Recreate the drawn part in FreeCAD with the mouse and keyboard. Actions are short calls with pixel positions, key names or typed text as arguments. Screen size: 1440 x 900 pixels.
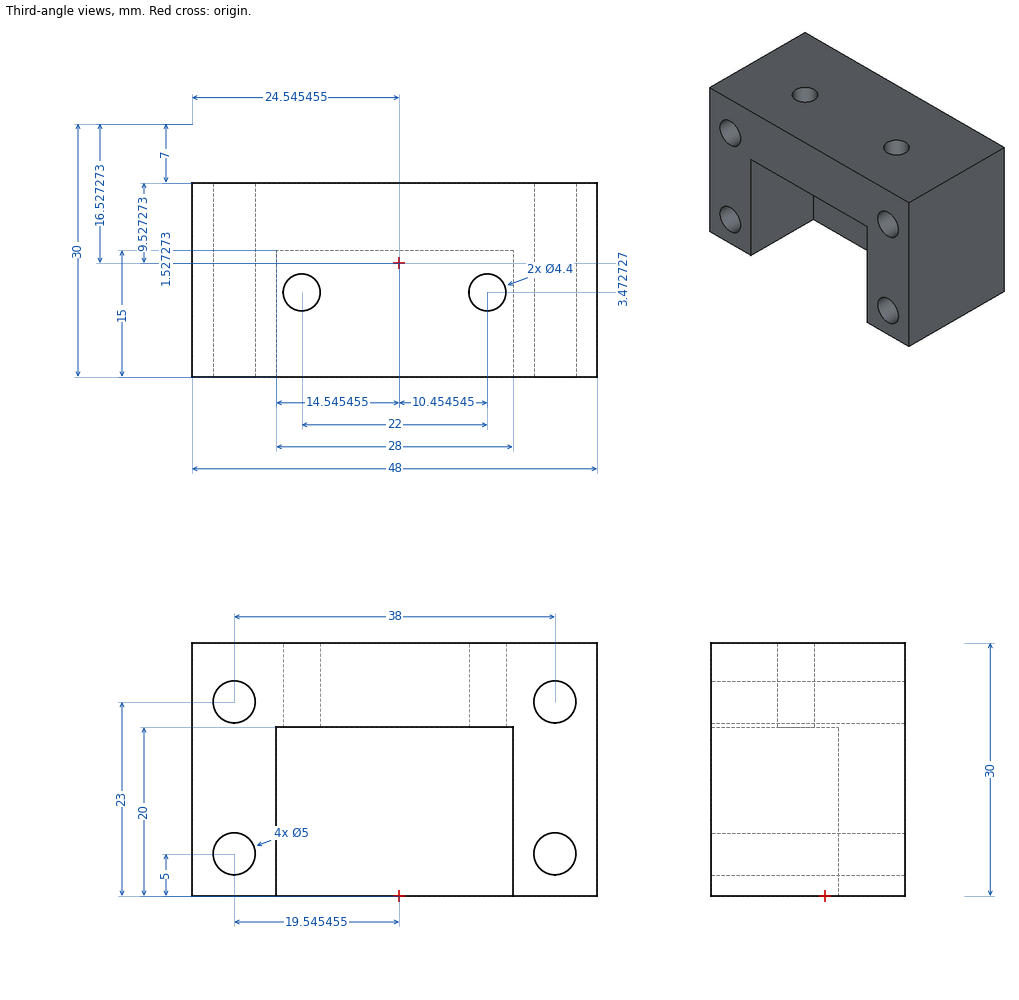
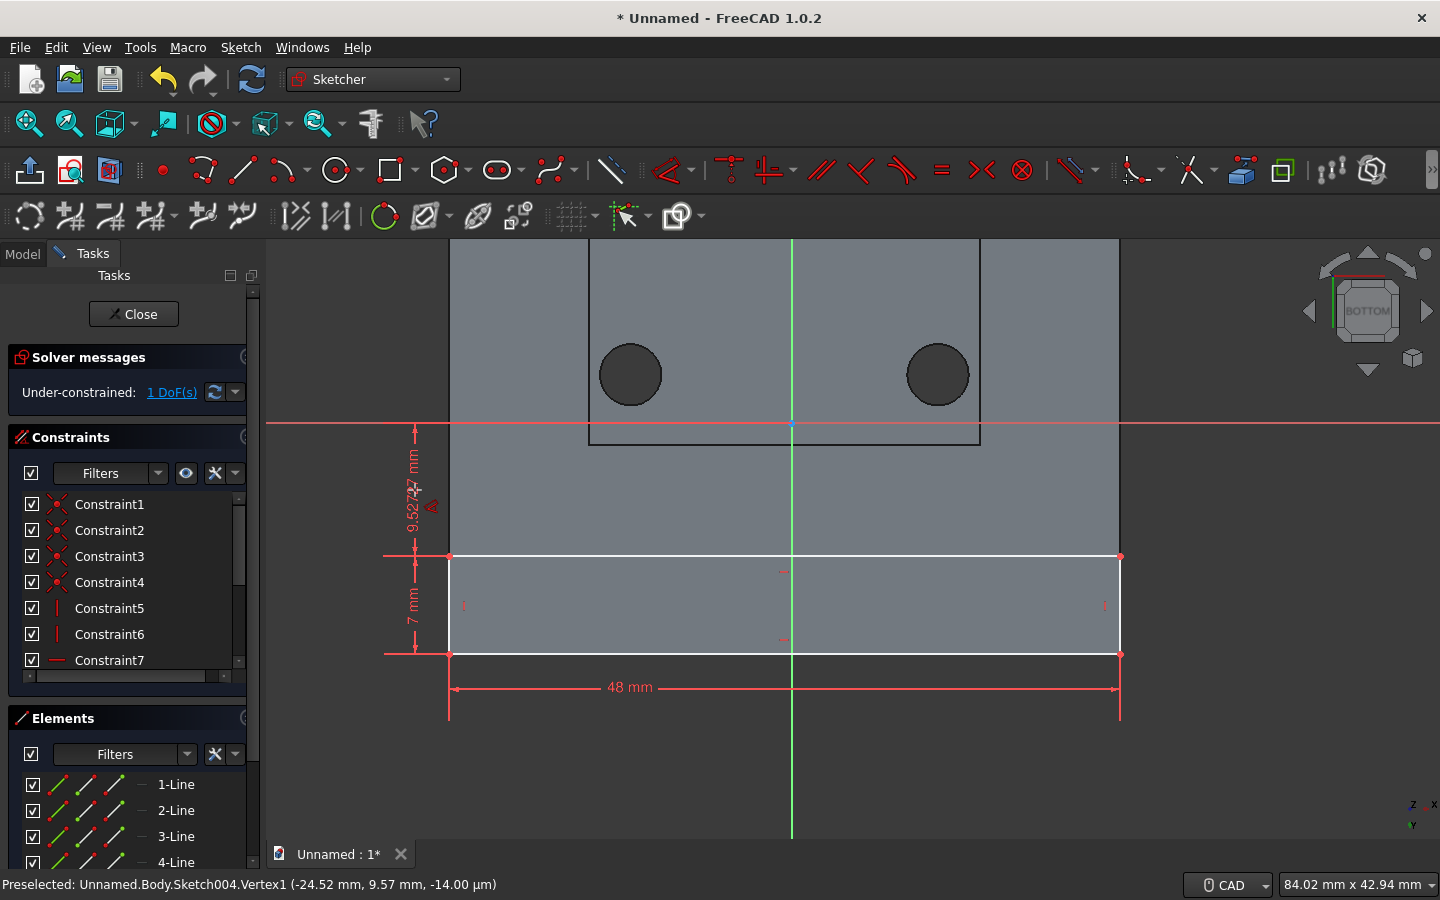
click(449, 556)
click(621, 389)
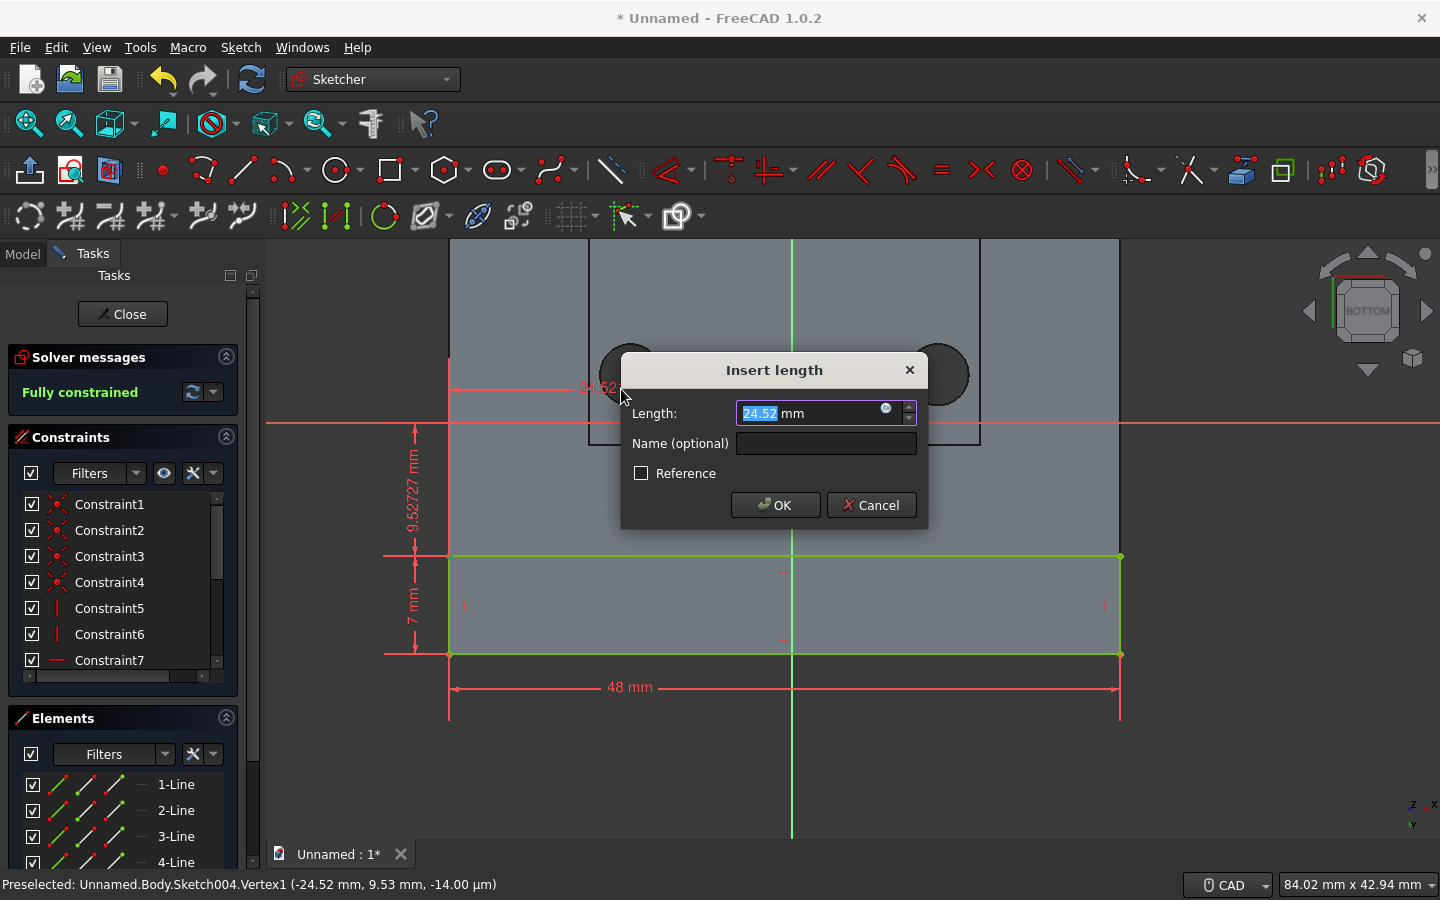
text(24.545455)
key(Return)
key(Escape)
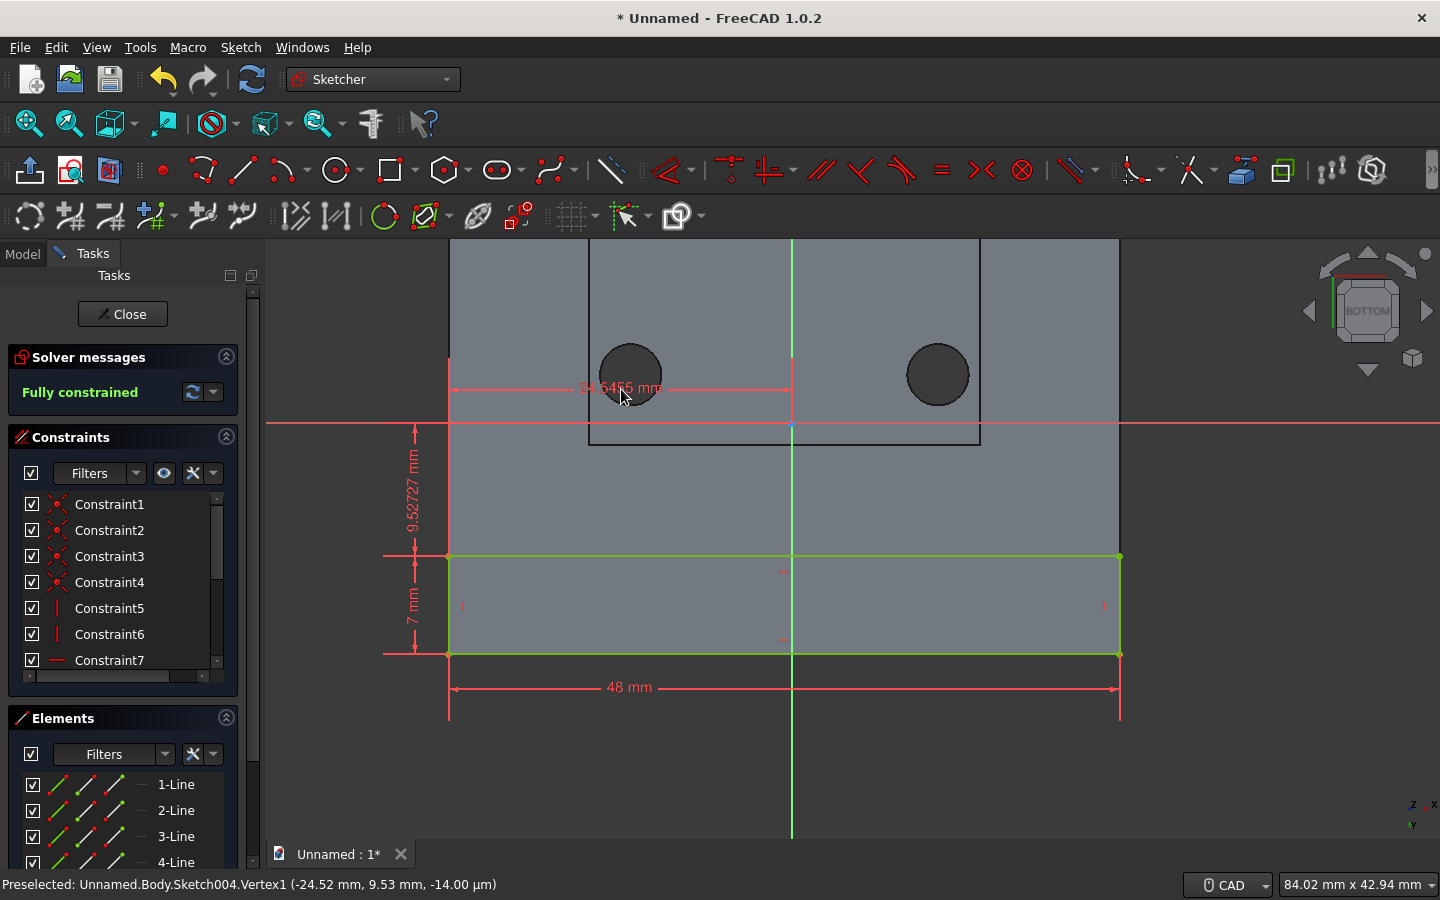
click(123, 314)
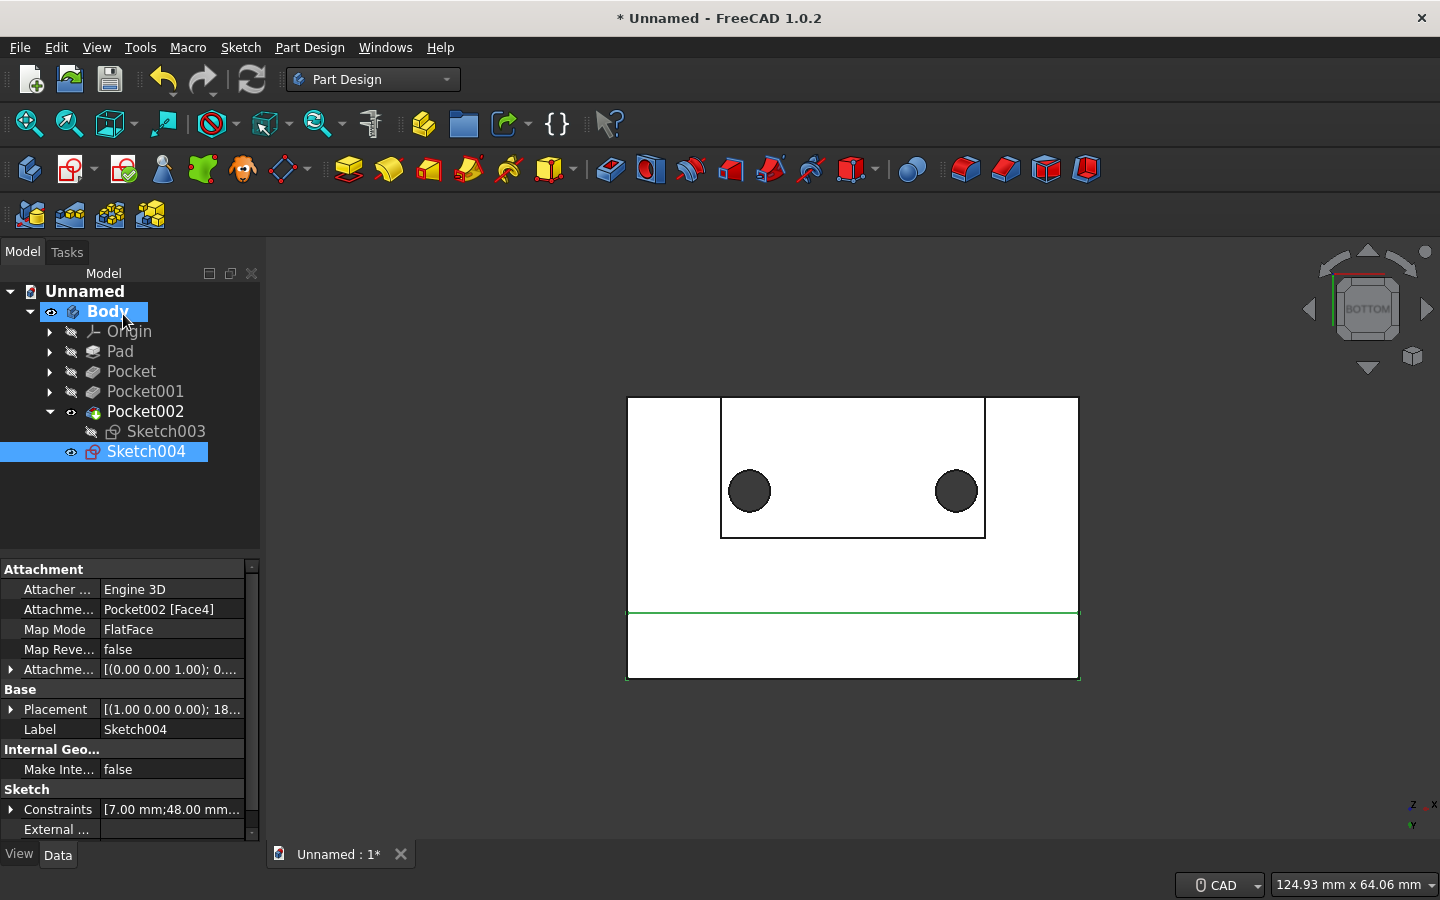
click(612, 170)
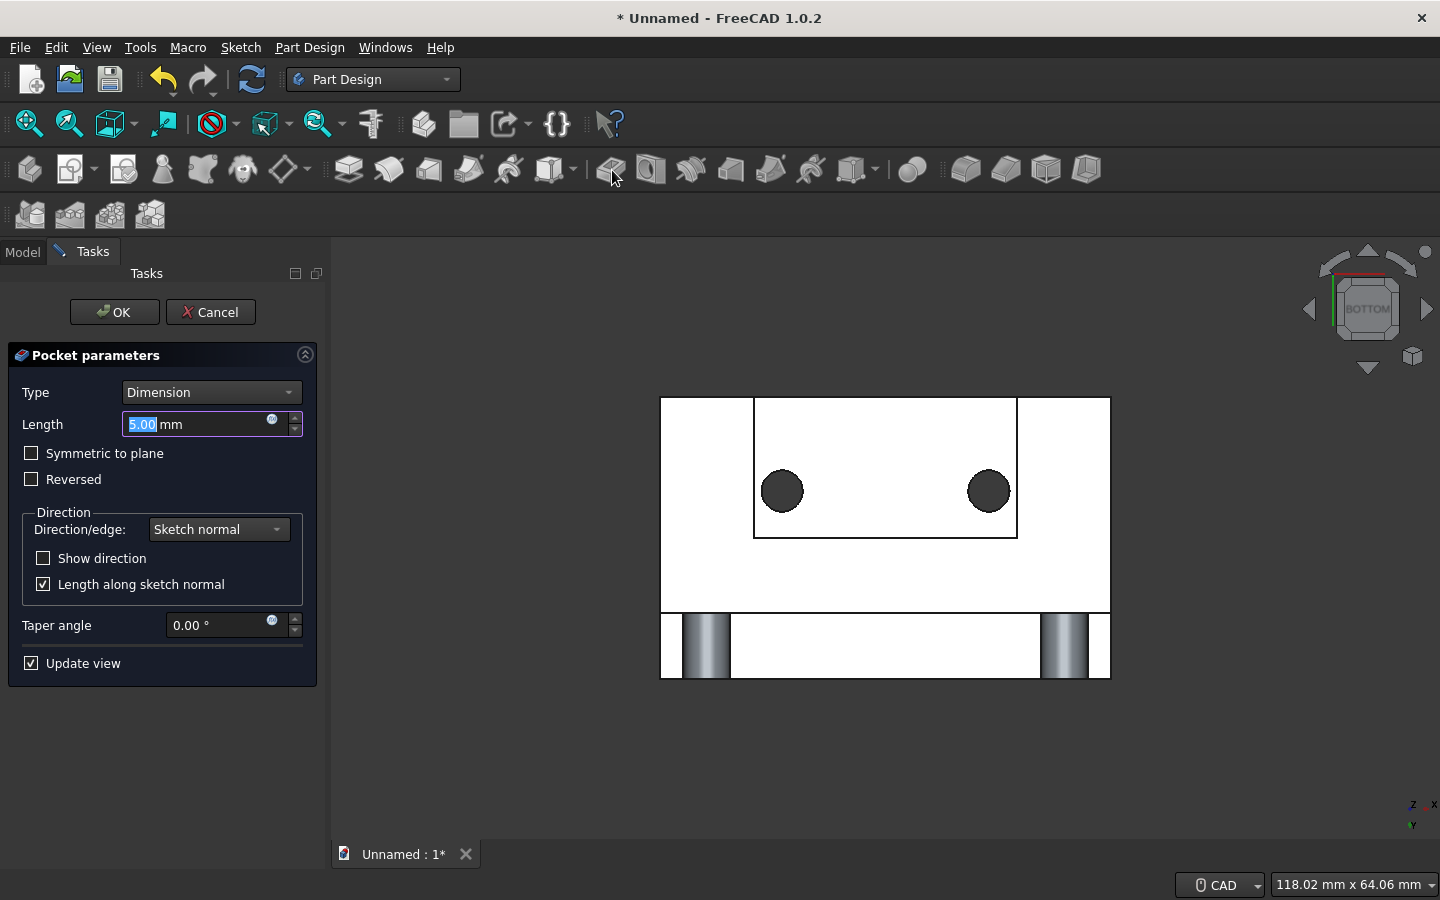
text(30)
key(Tab)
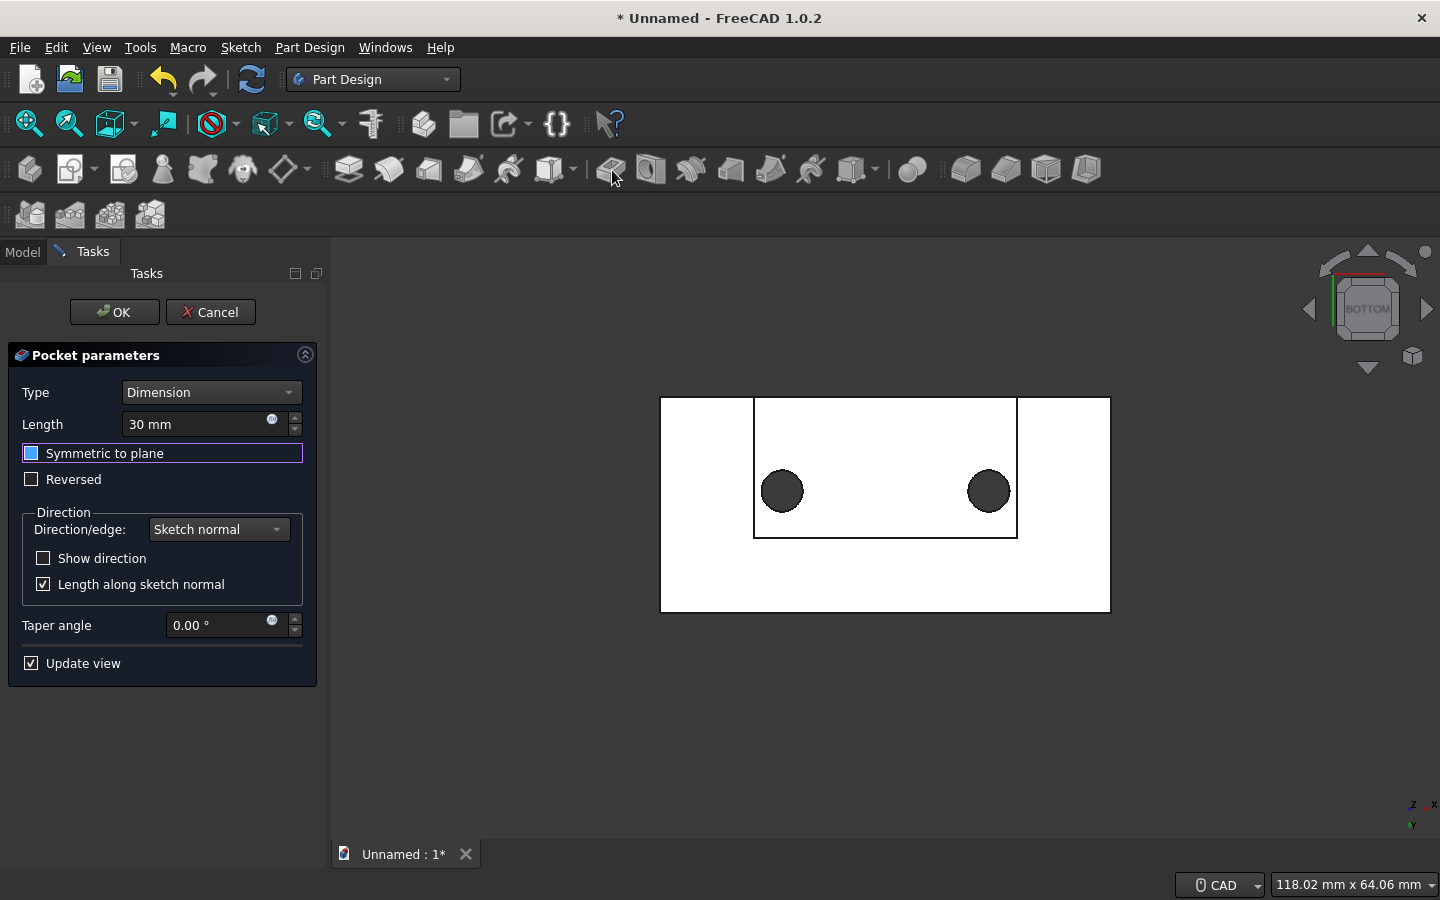
click(115, 312)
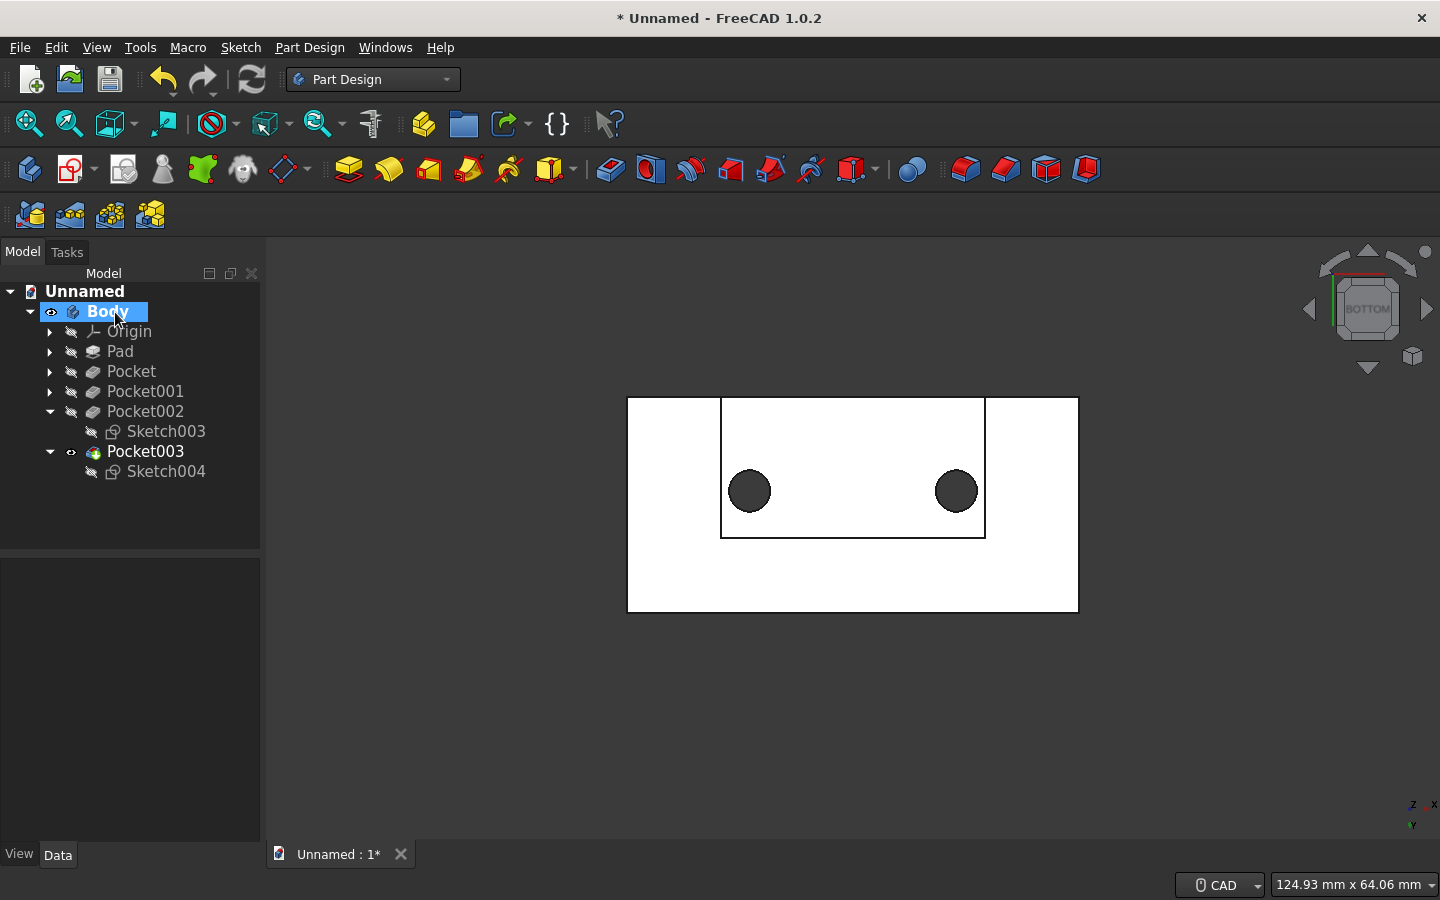
key(0)